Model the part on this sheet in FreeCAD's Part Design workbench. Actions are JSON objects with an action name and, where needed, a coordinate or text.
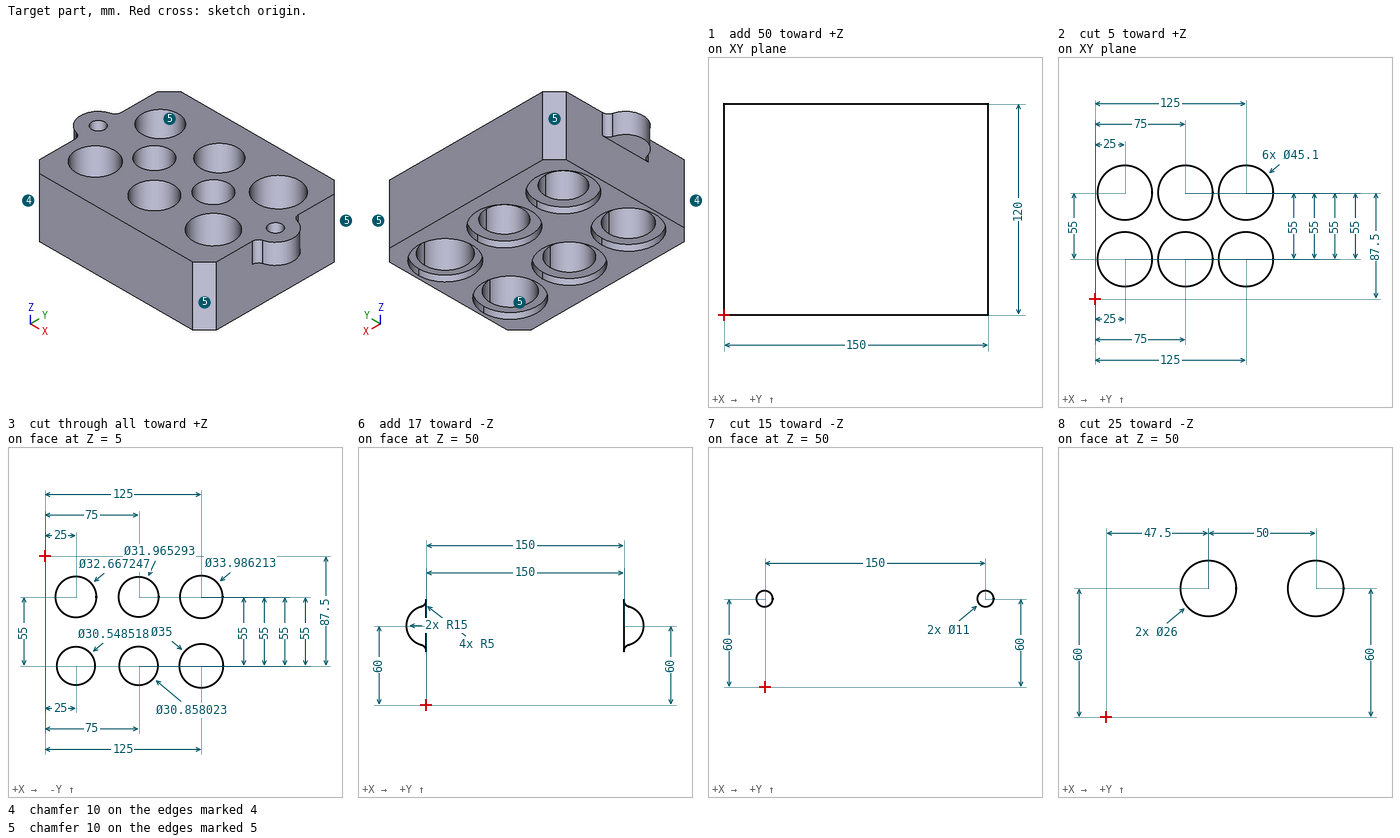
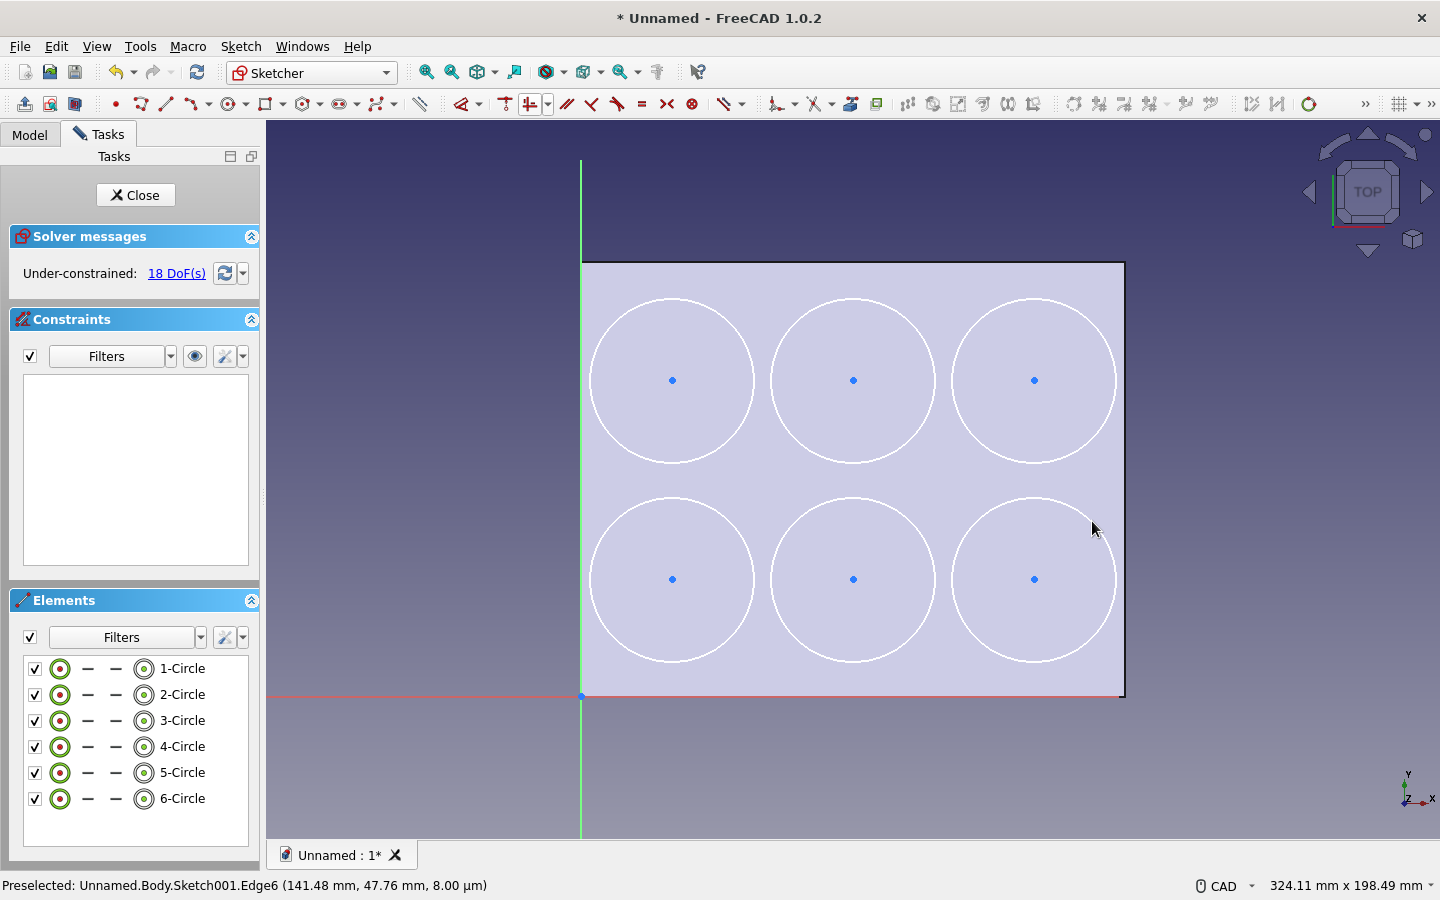
{"action": "left_click", "coordinate": [1092, 323]}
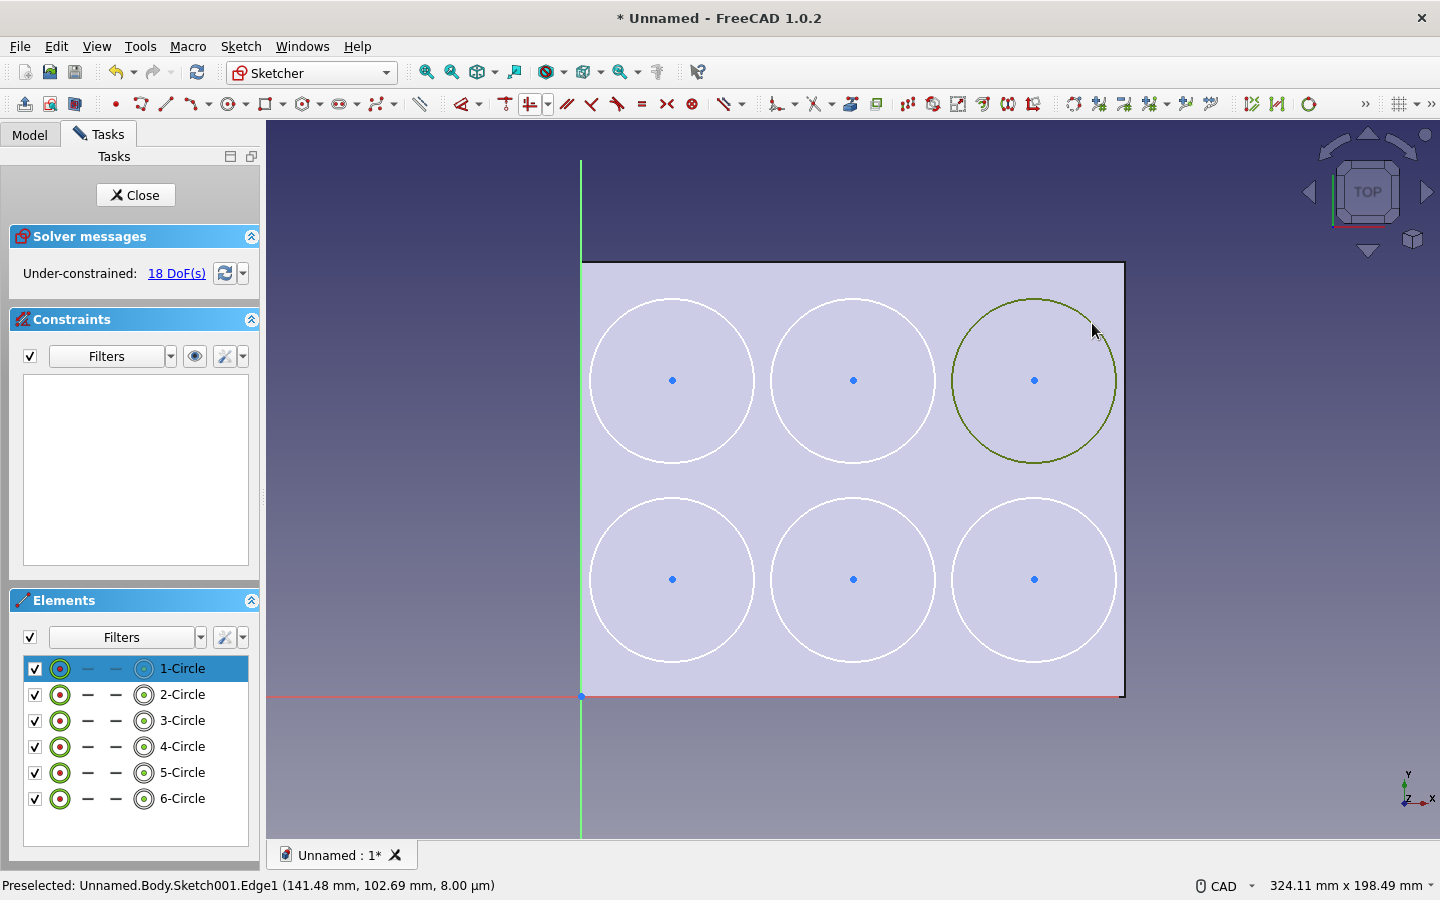
{"action": "left_click", "coordinate": [911, 323]}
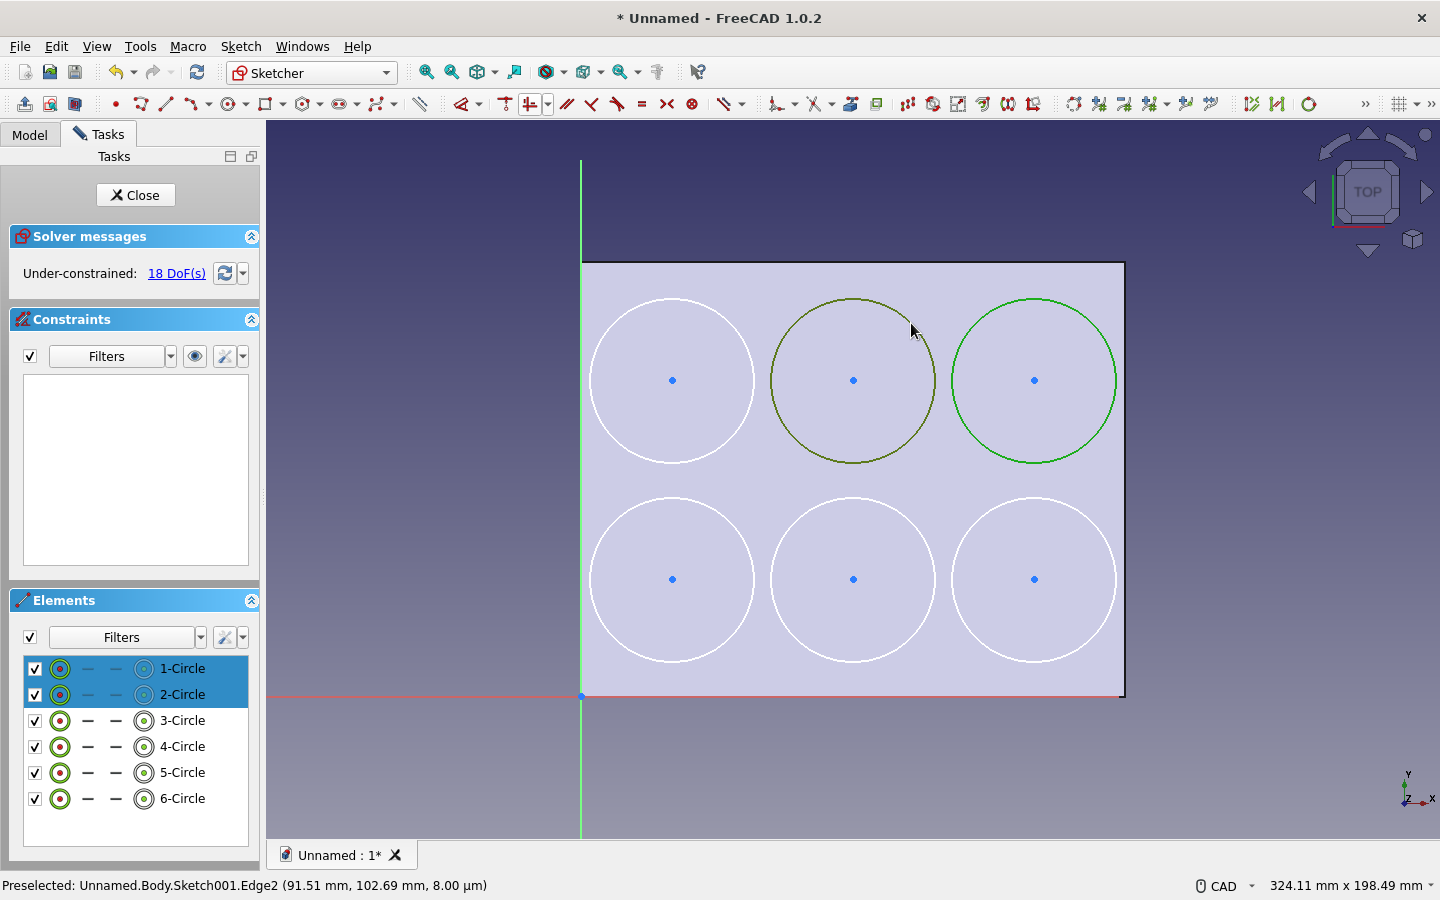
{"action": "left_click", "coordinate": [730, 323]}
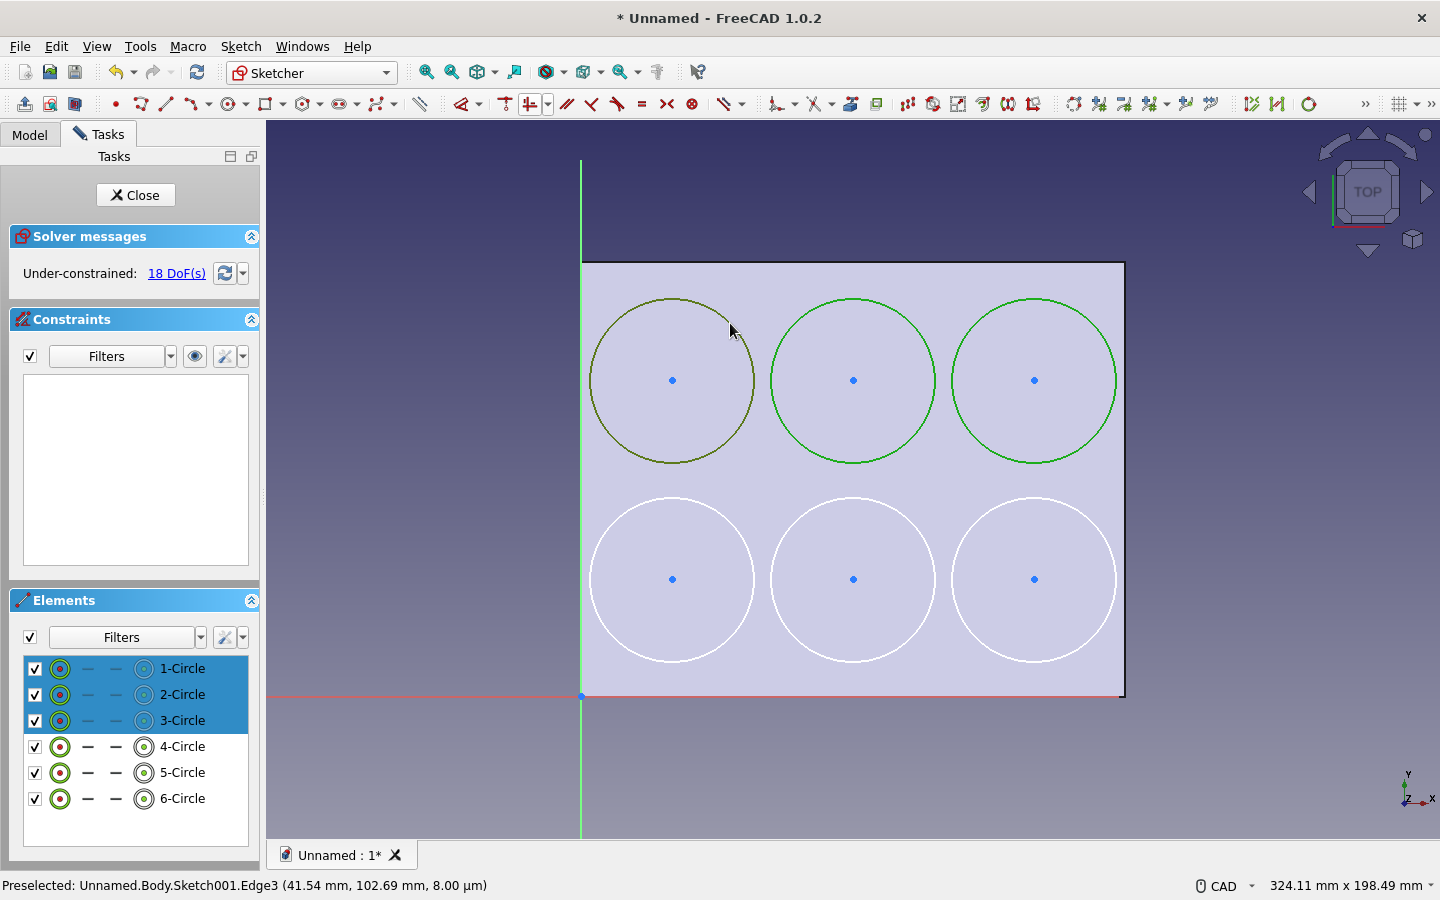
{"action": "left_click", "coordinate": [730, 522]}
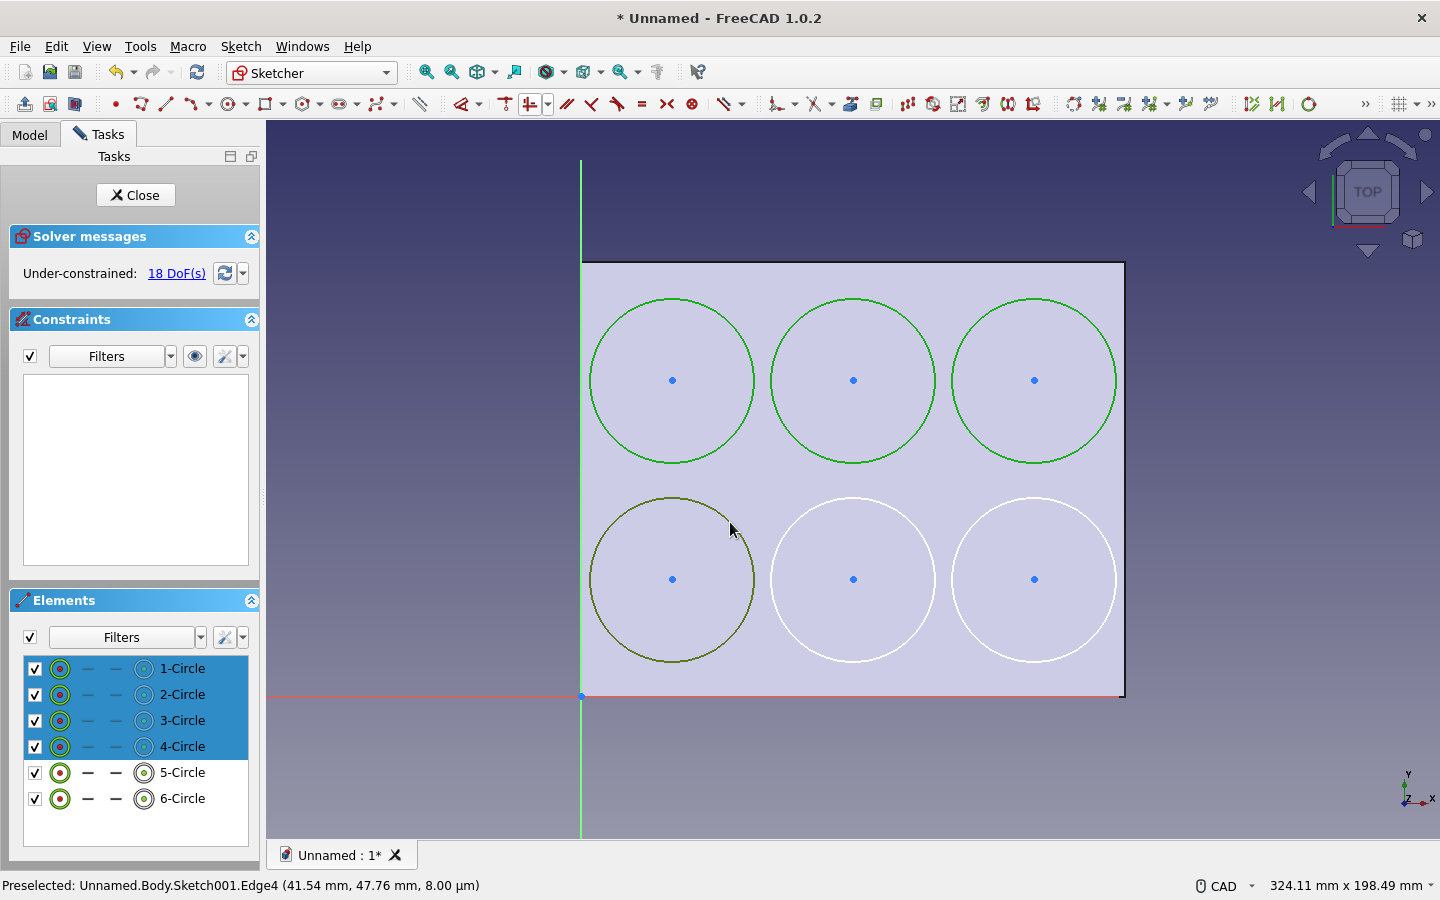
{"action": "left_click", "coordinate": [911, 522]}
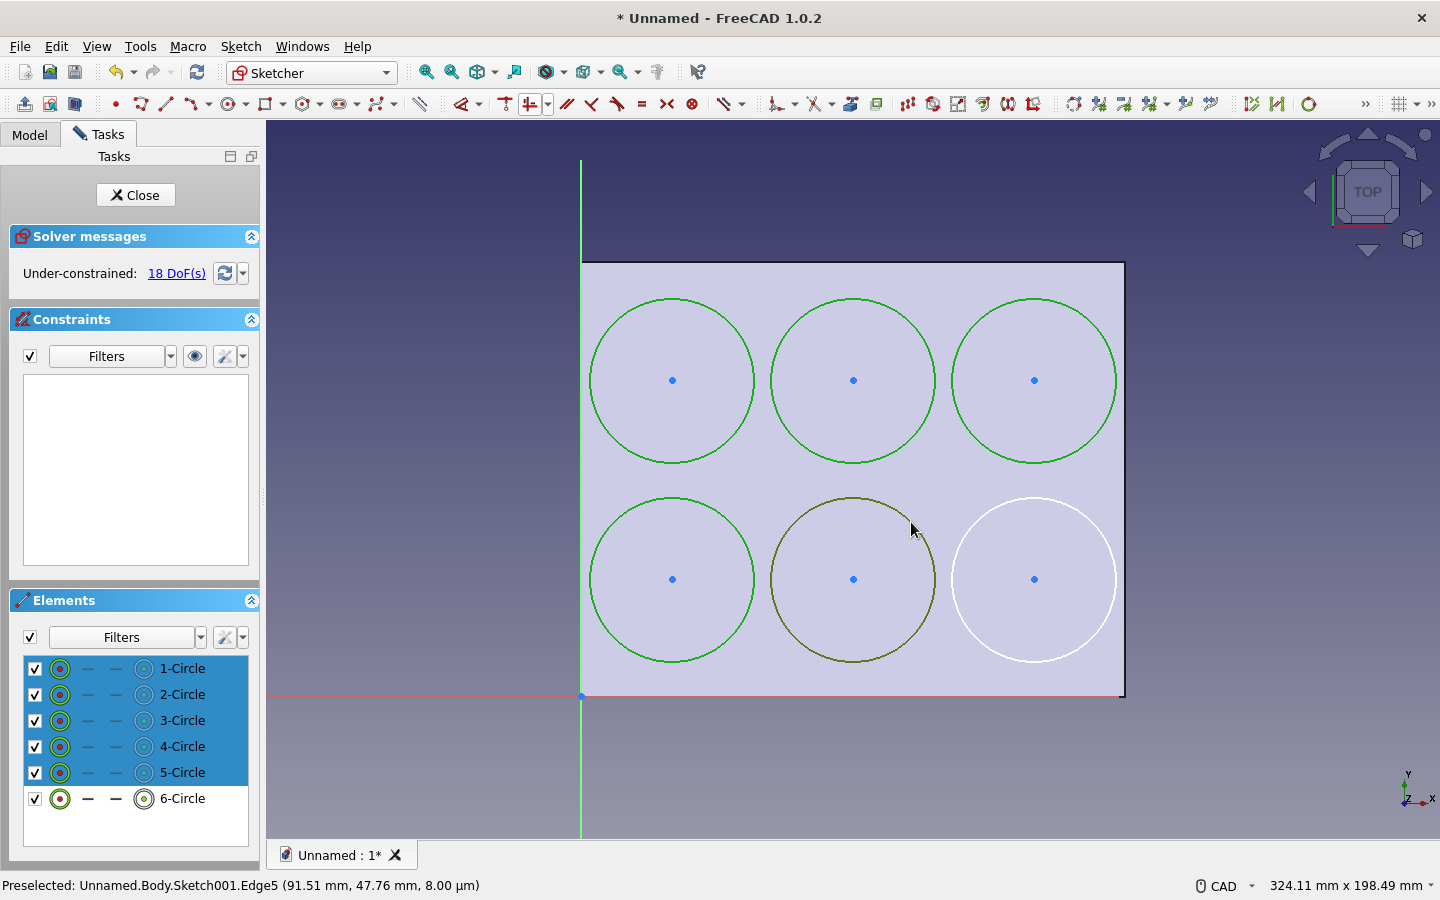
{"action": "left_click", "coordinate": [1092, 522]}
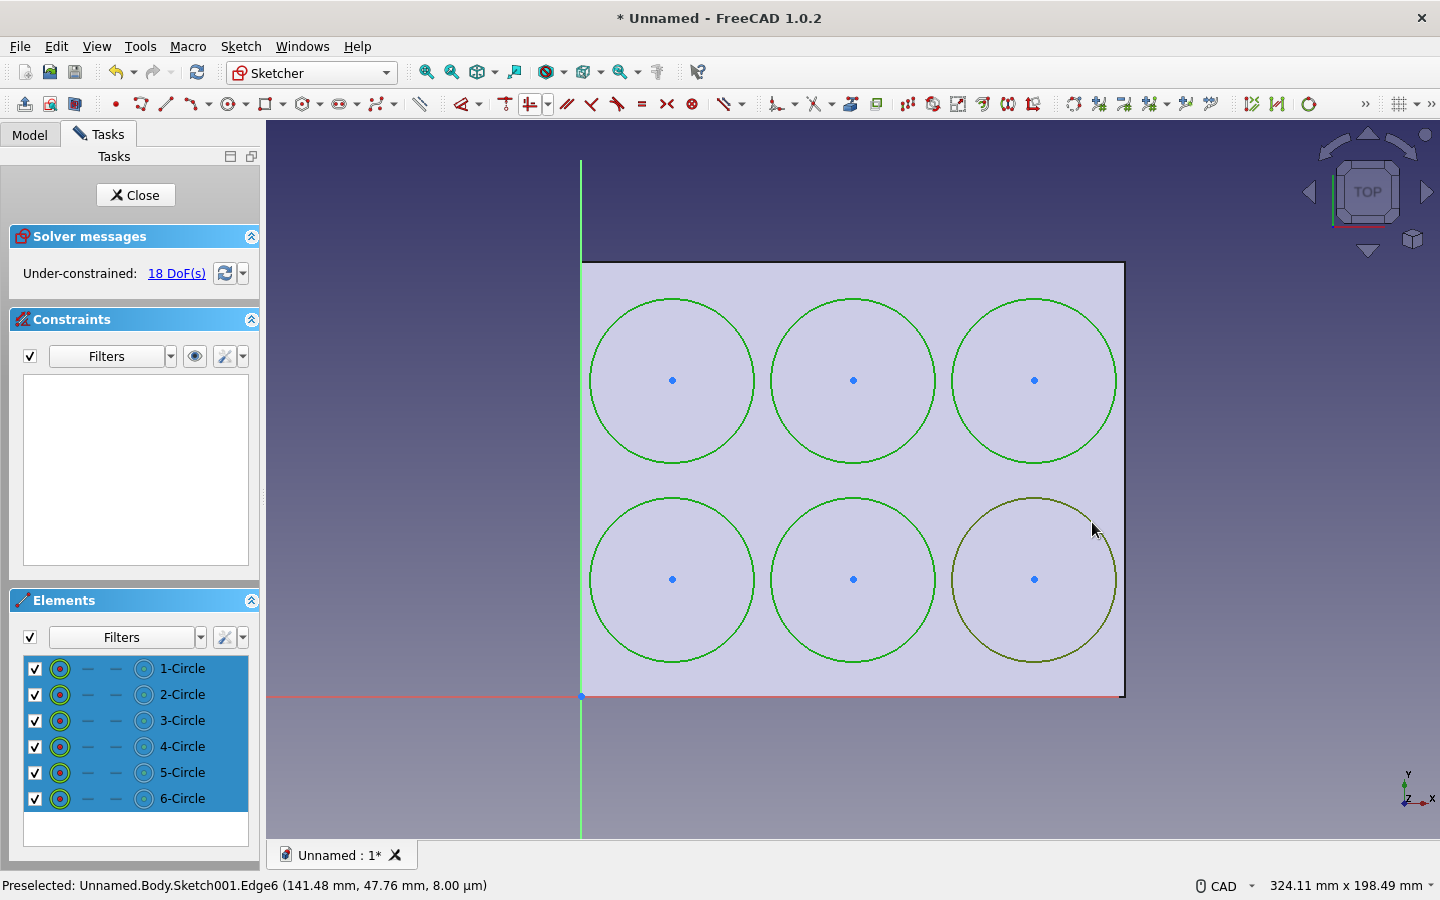
{"action": "left_click", "coordinate": [642, 104]}